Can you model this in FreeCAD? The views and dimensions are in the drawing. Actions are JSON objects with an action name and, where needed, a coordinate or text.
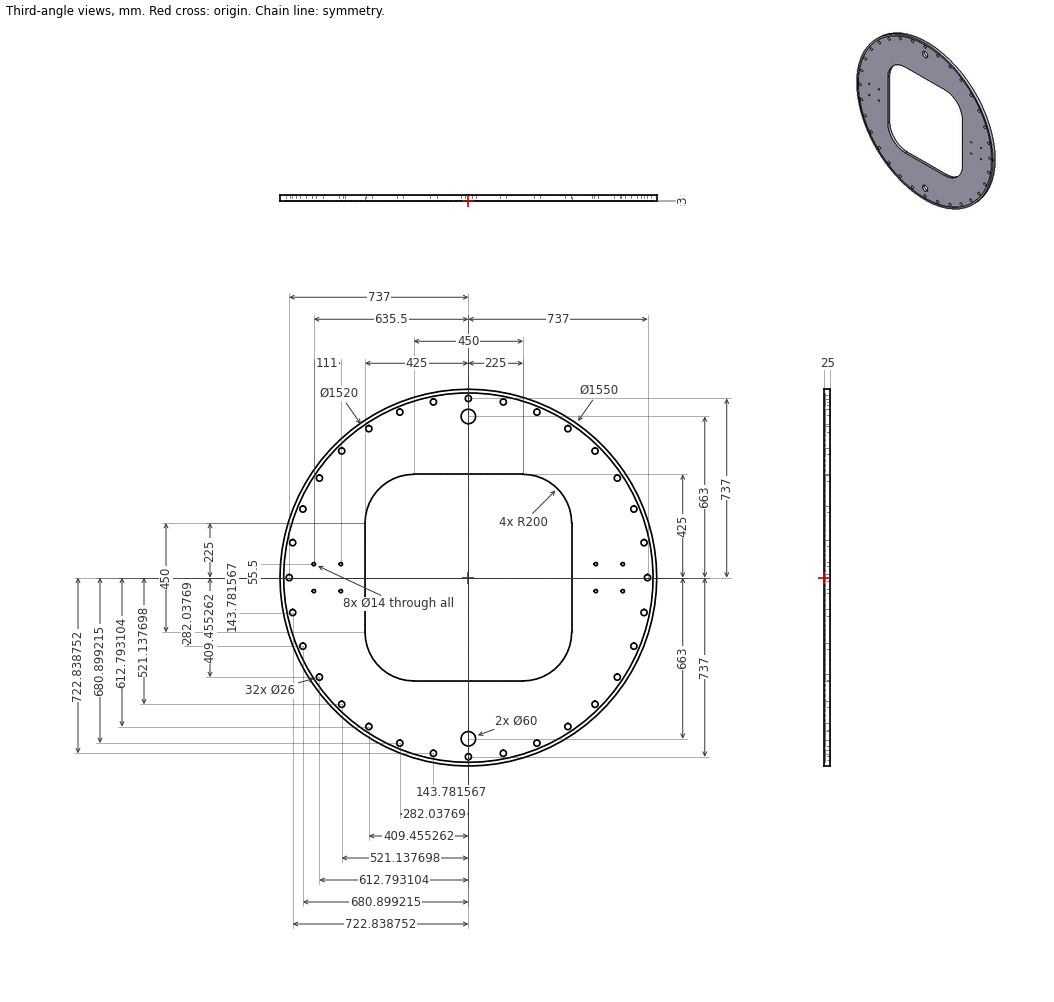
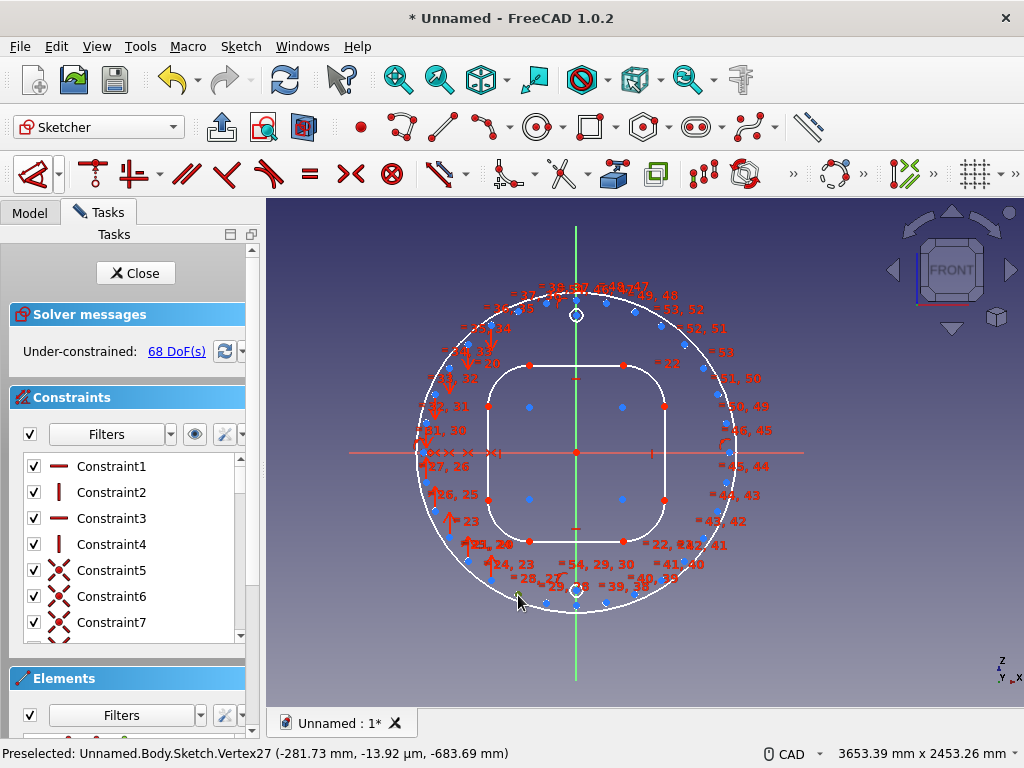
{"action": "left_click", "coordinate": [518, 312]}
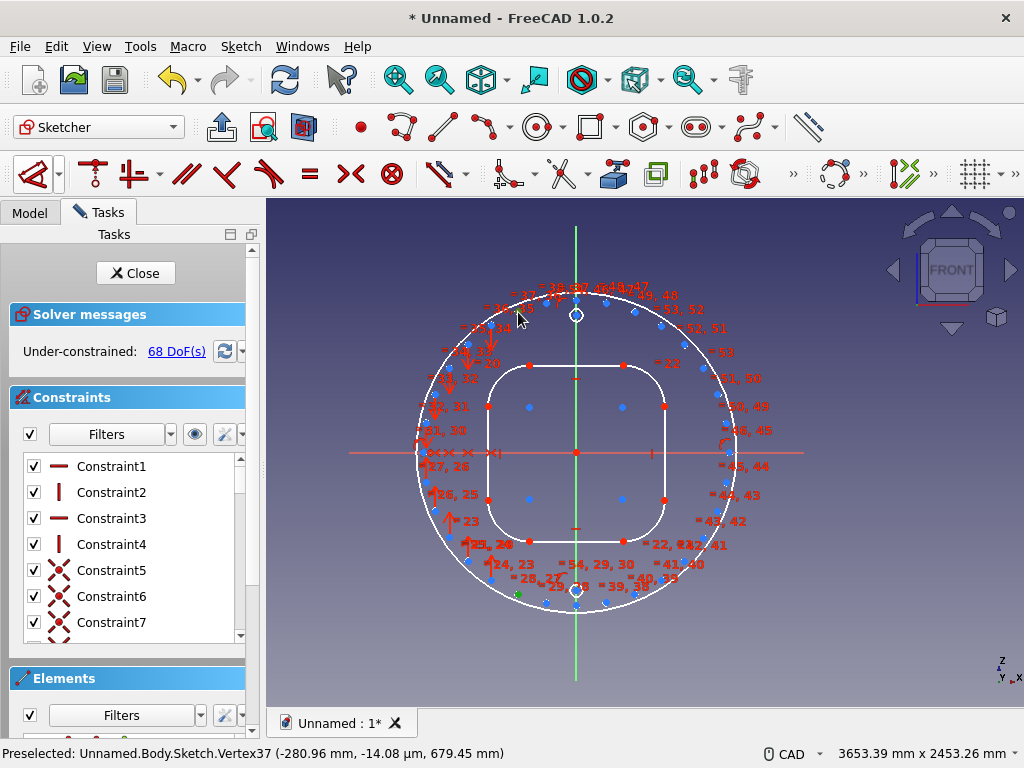
{"action": "left_click", "coordinate": [375, 453]}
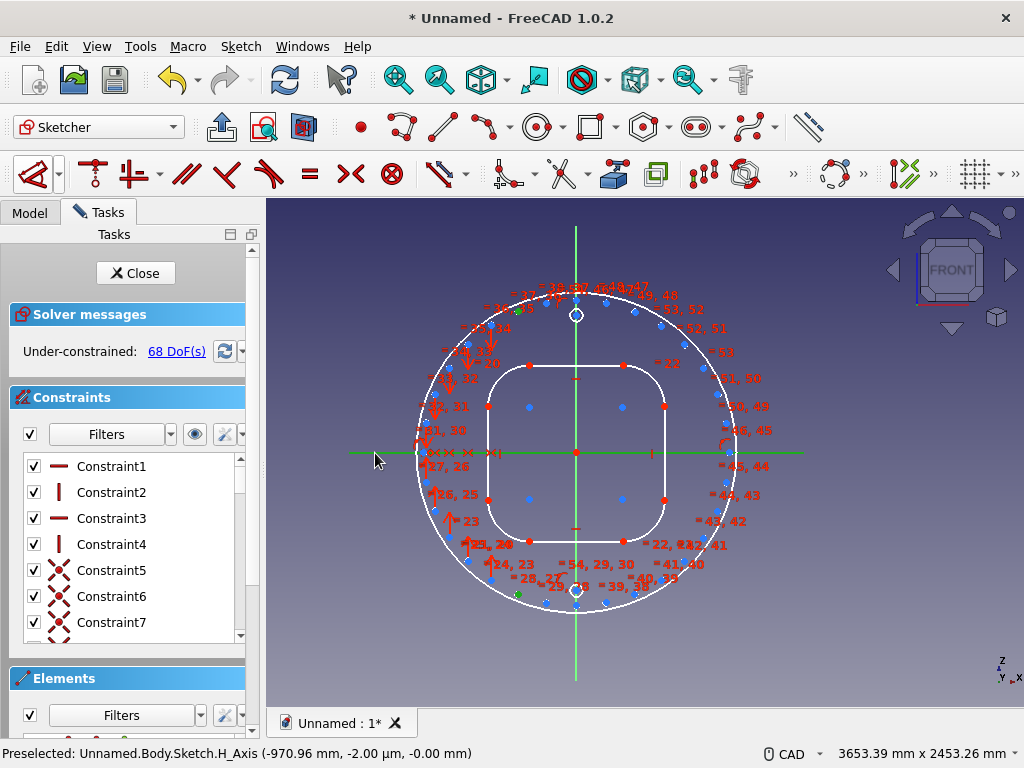
{"action": "left_click", "coordinate": [351, 174]}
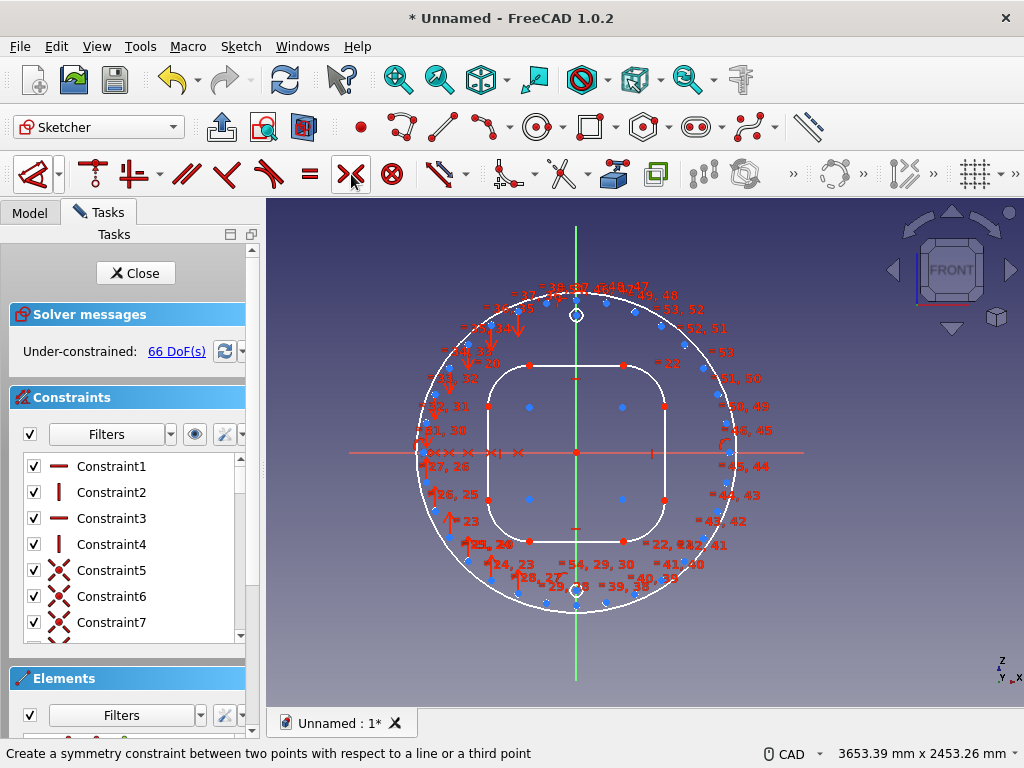
{"action": "left_click", "coordinate": [547, 603]}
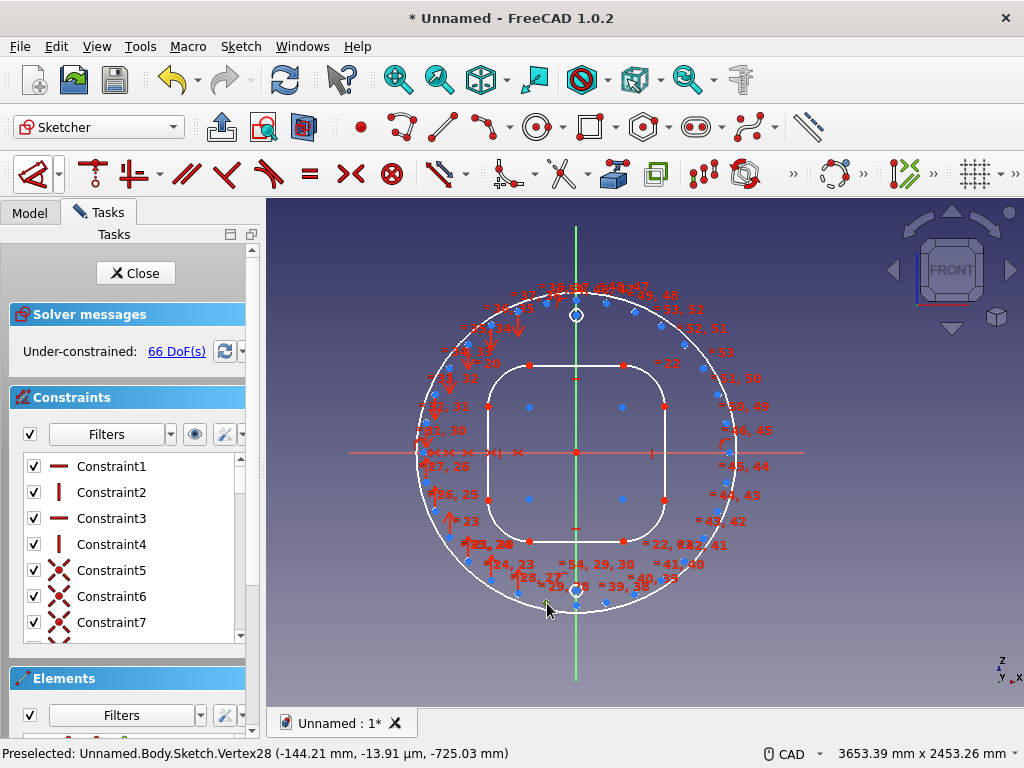
{"action": "left_click", "coordinate": [547, 303]}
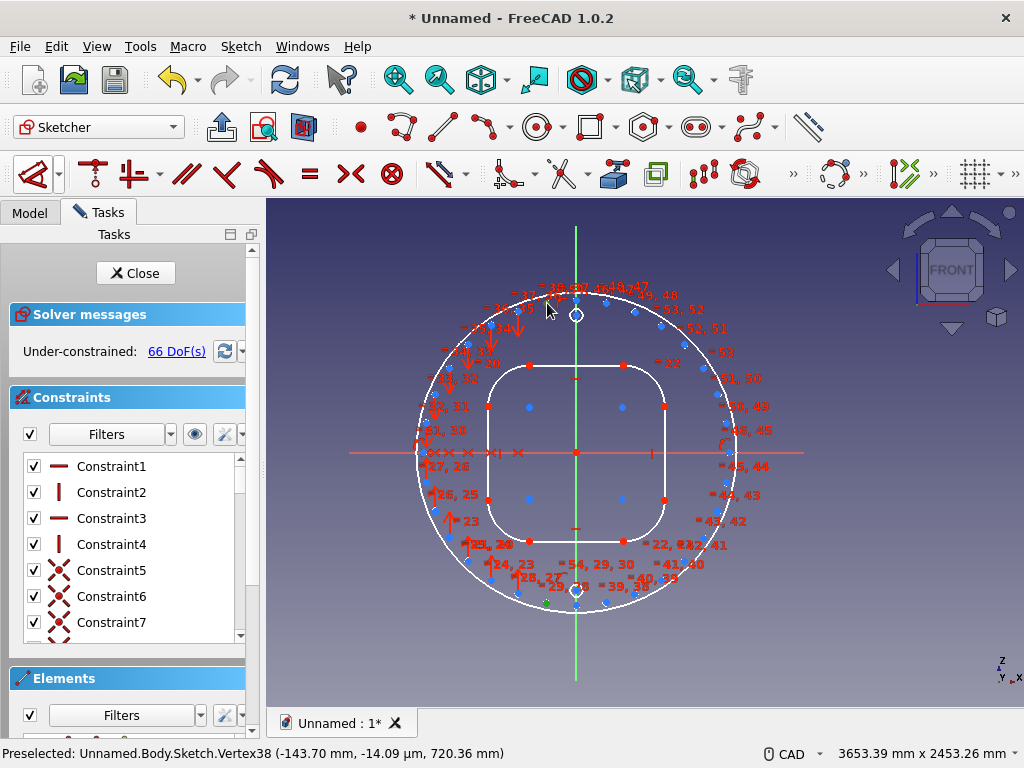
{"action": "left_click", "coordinate": [375, 453]}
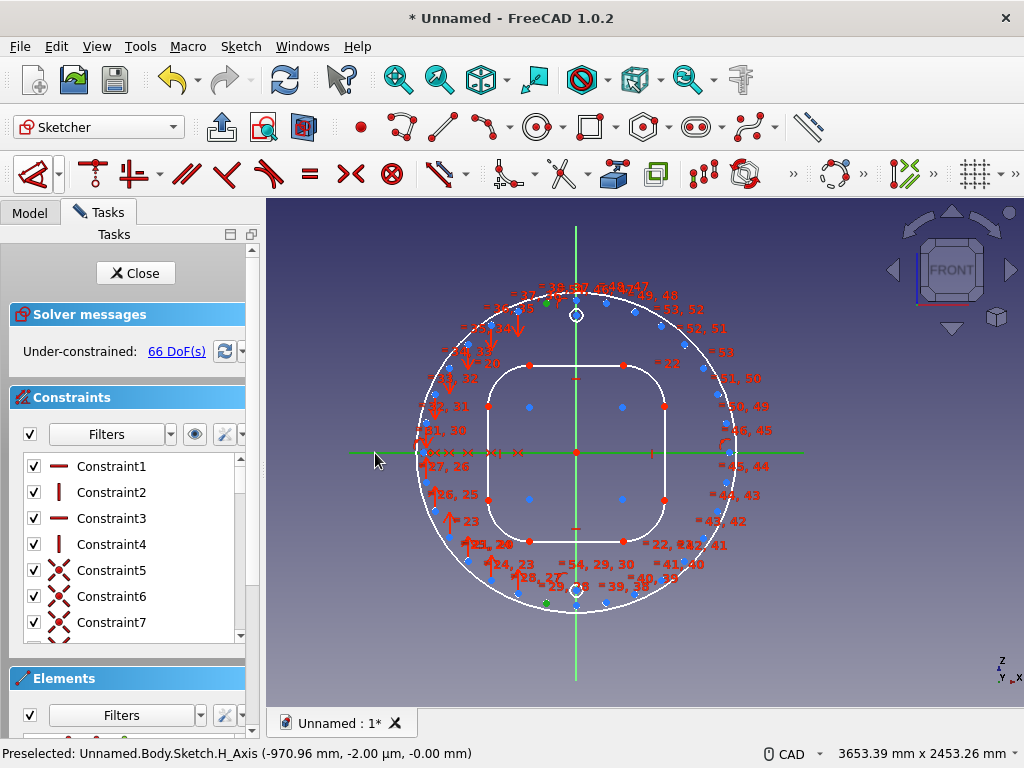
{"action": "left_click", "coordinate": [351, 174]}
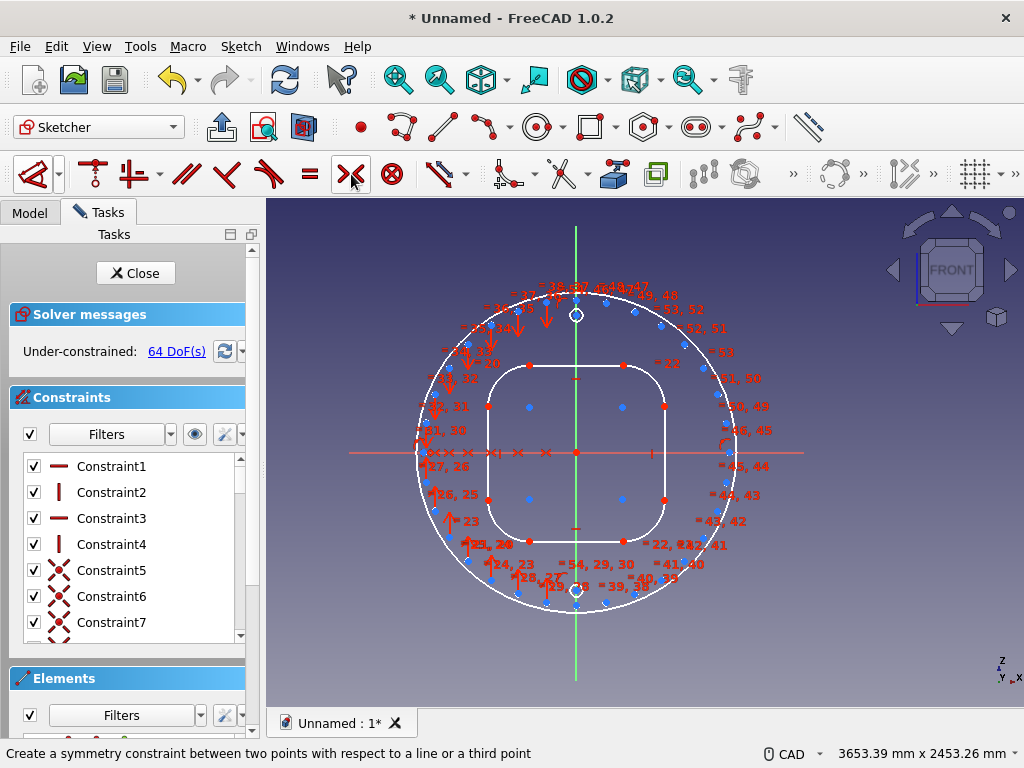
{"action": "left_click", "coordinate": [547, 603]}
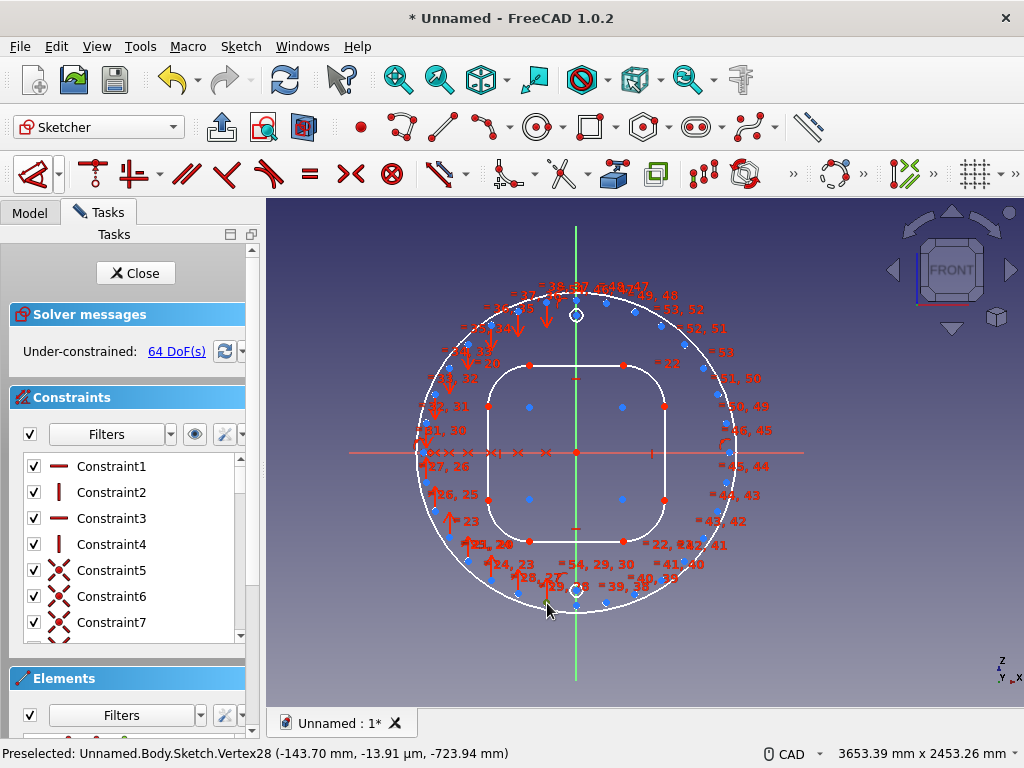
{"action": "left_click", "coordinate": [606, 603]}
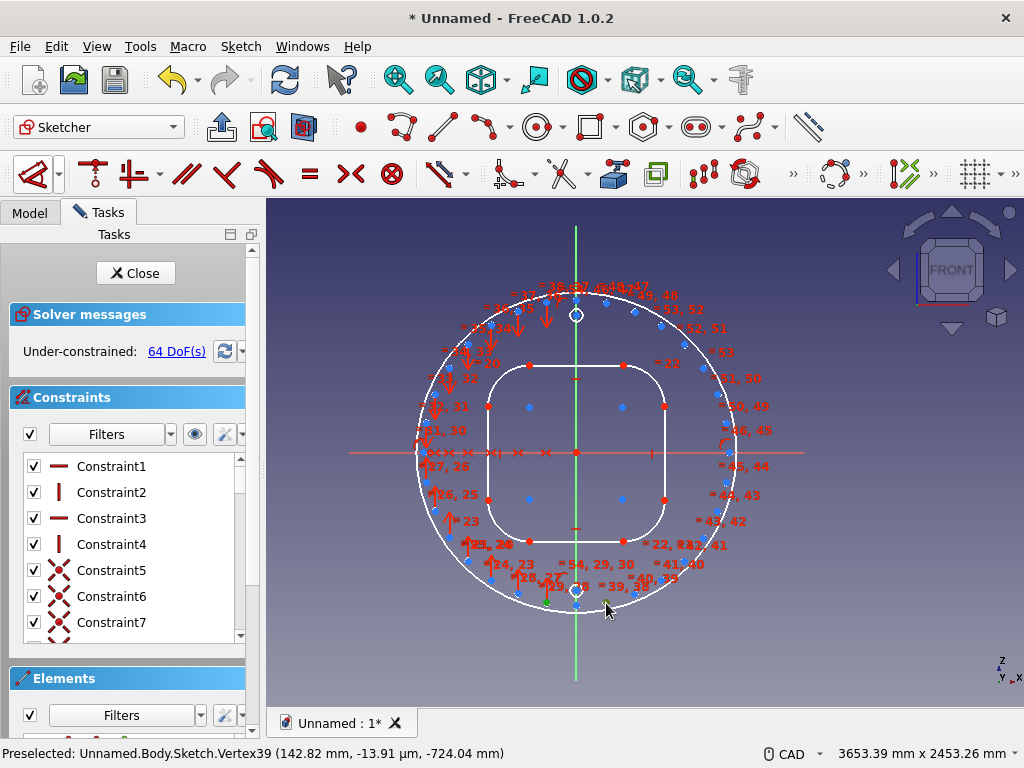
{"action": "left_click", "coordinate": [576, 647]}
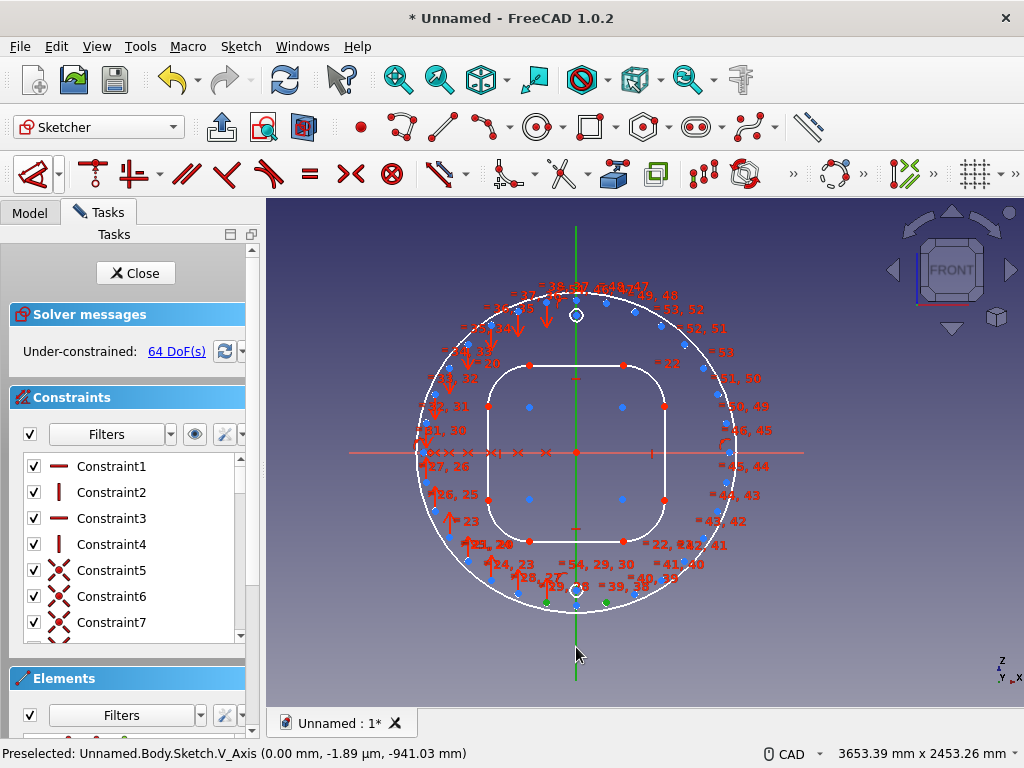
{"action": "left_click", "coordinate": [351, 174]}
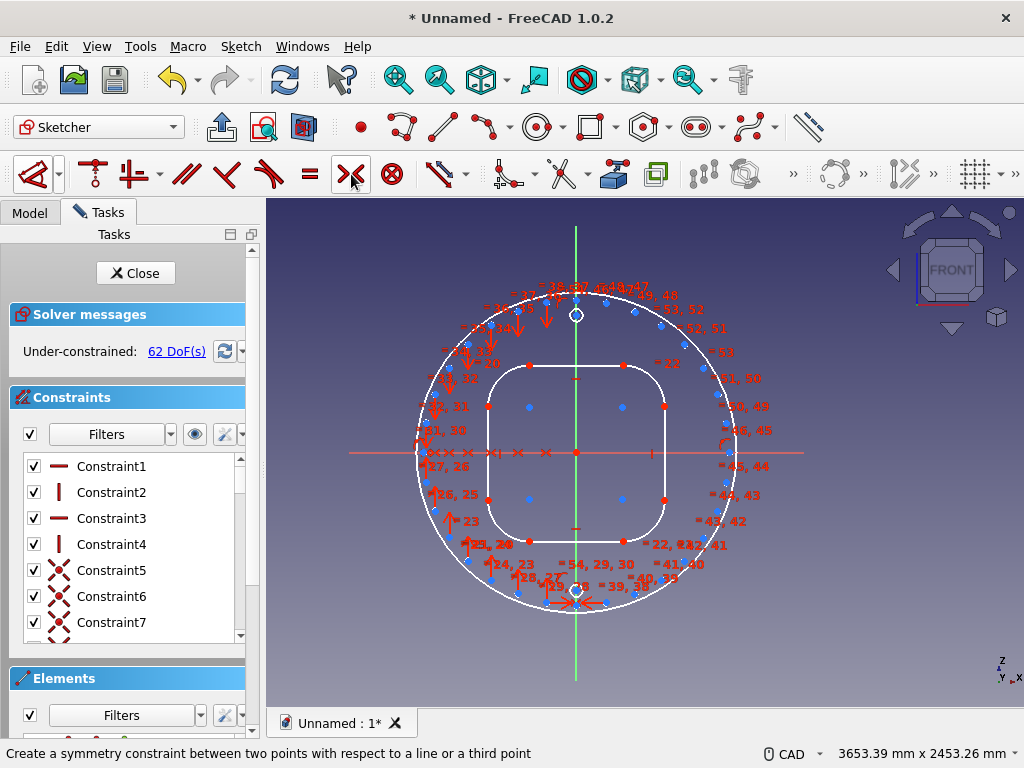
{"action": "left_click", "coordinate": [518, 594]}